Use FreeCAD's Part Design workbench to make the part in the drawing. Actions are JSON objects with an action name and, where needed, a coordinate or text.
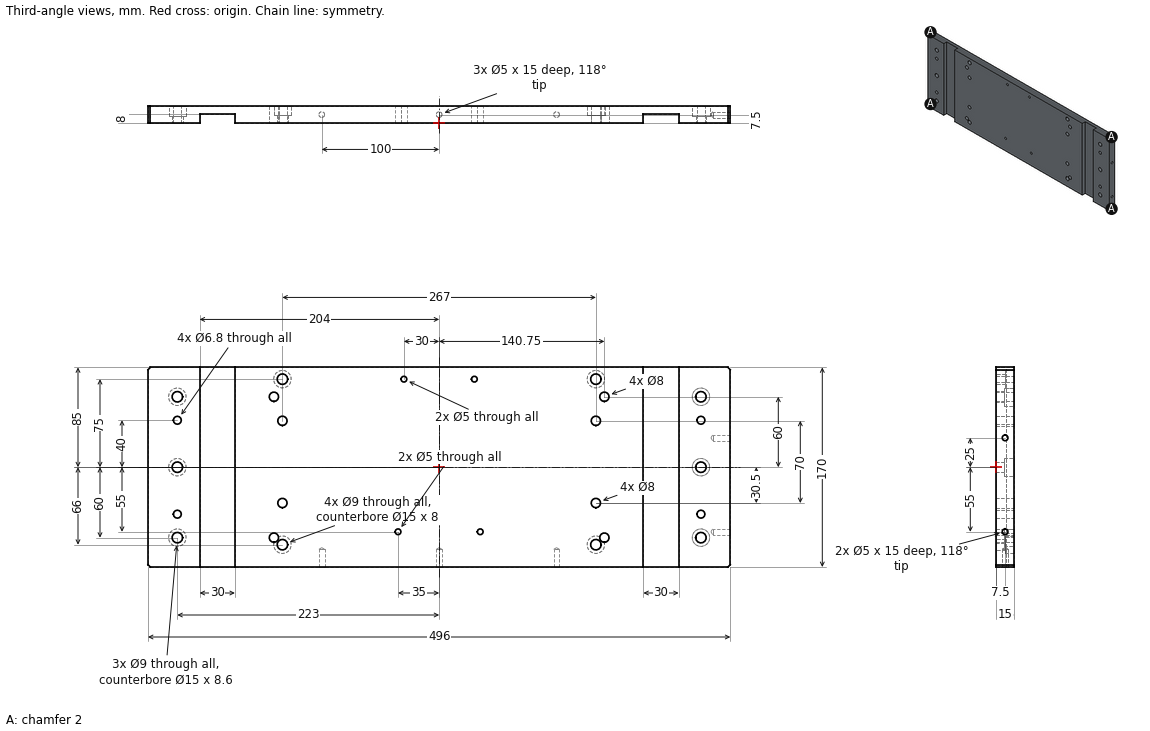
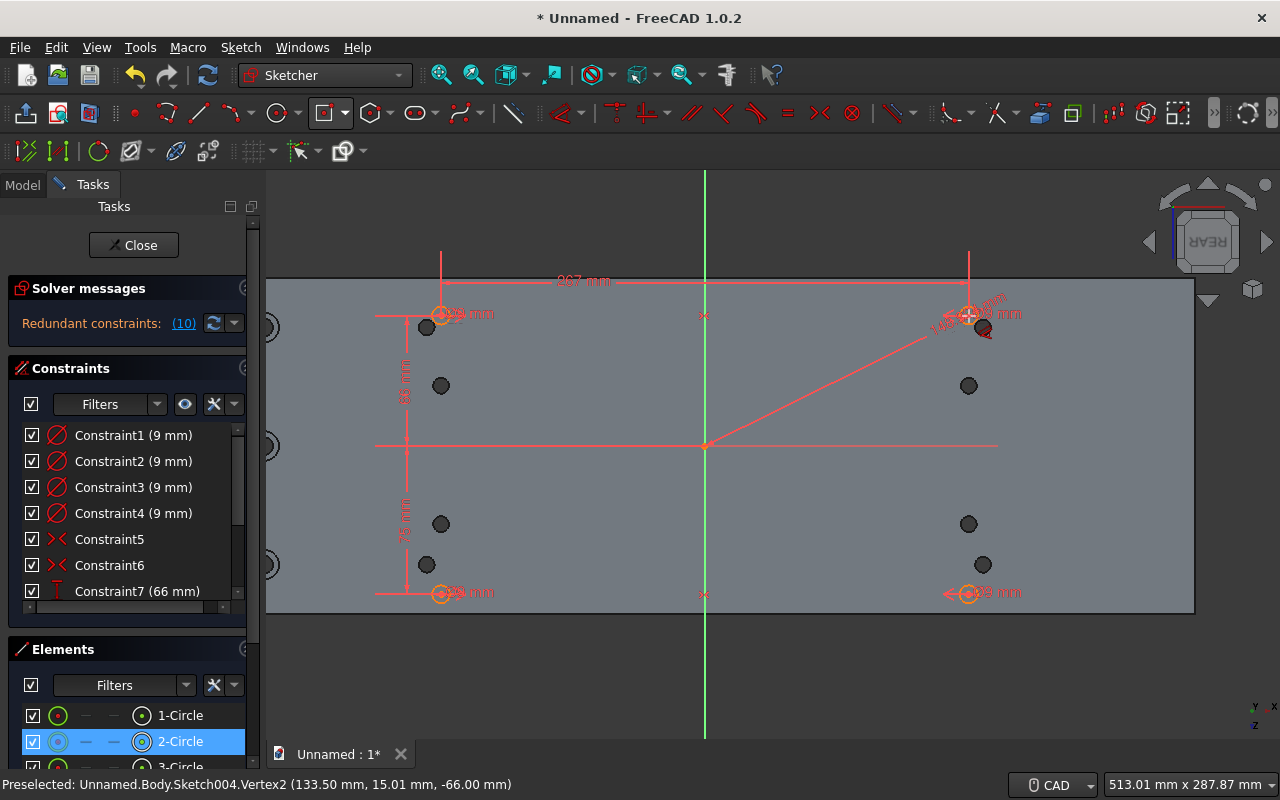
{"action": "left_click", "coordinate": [441, 594]}
{"action": "left_click", "coordinate": [584, 628]}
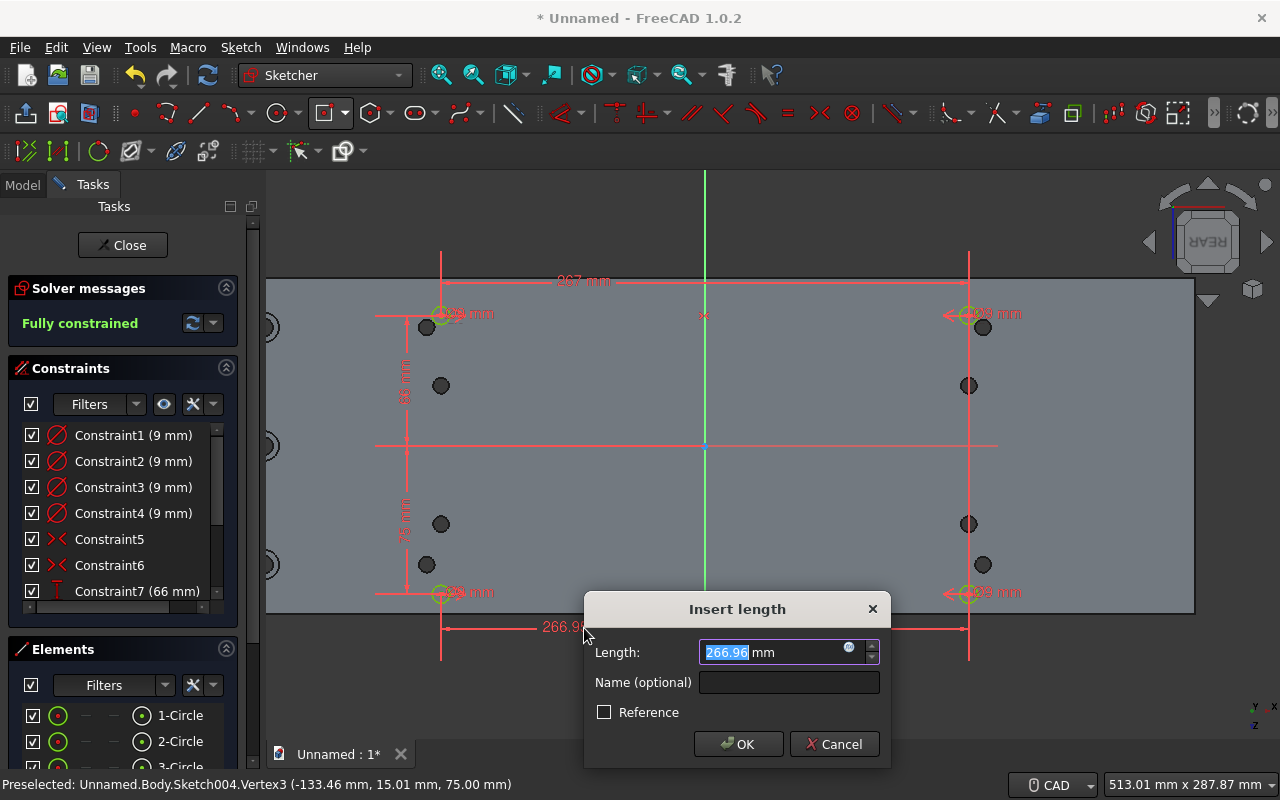
{"action": "type", "text": "267"}
{"action": "key", "text": "Return"}
{"action": "key", "text": "Escape"}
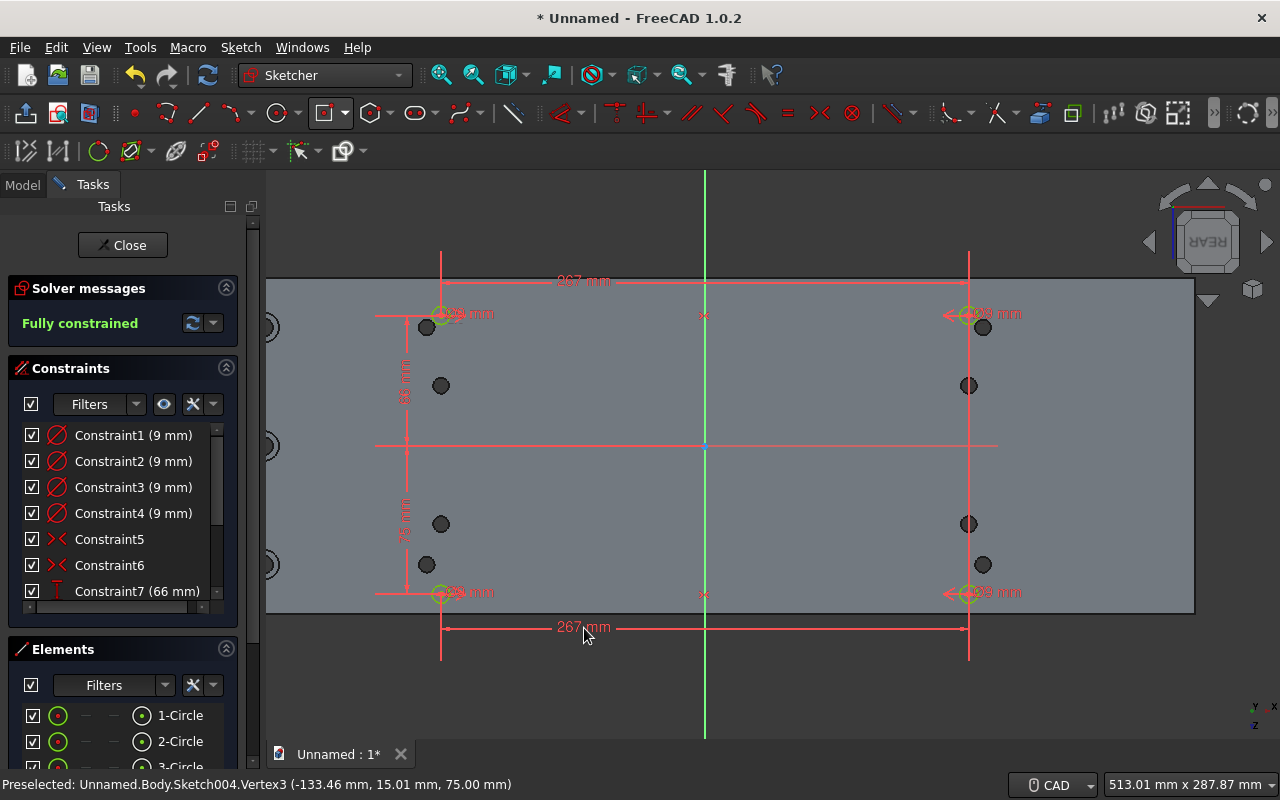
{"action": "left_click", "coordinate": [123, 245]}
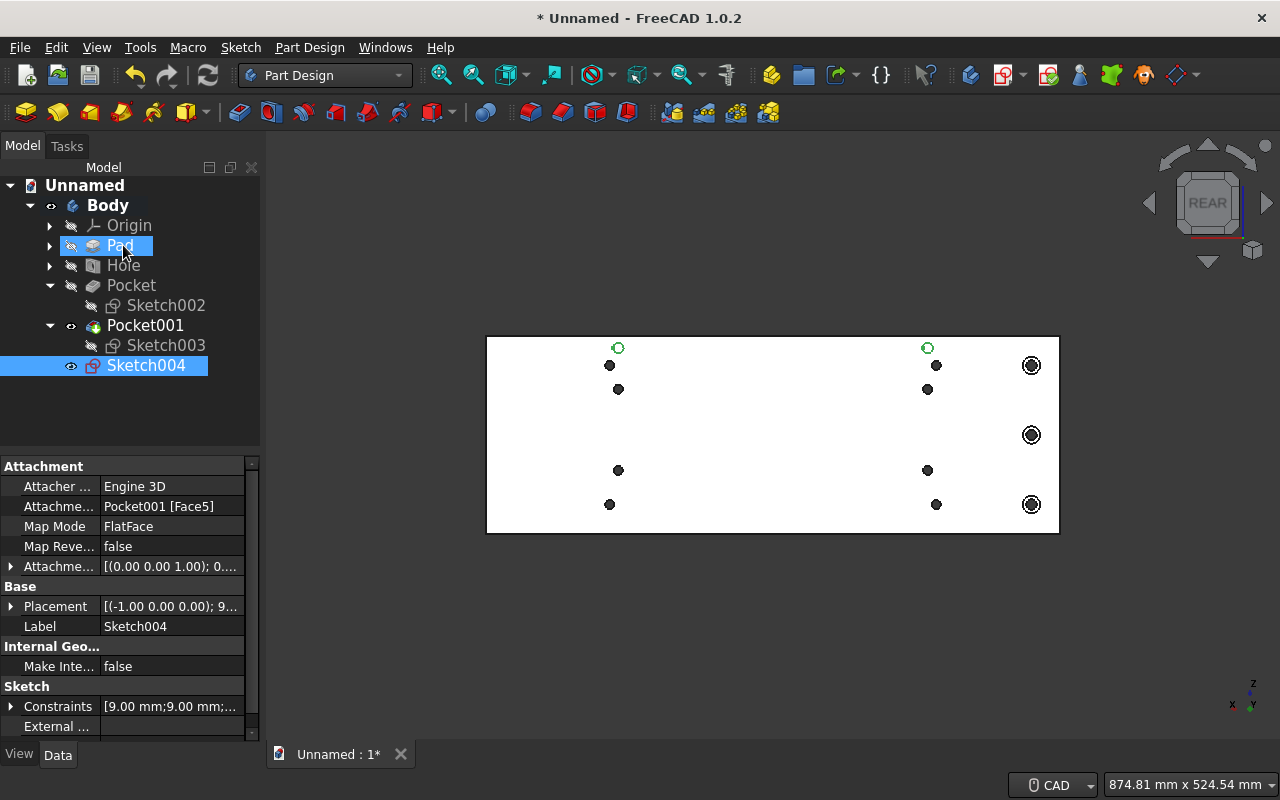
{"action": "left_click", "coordinate": [272, 112]}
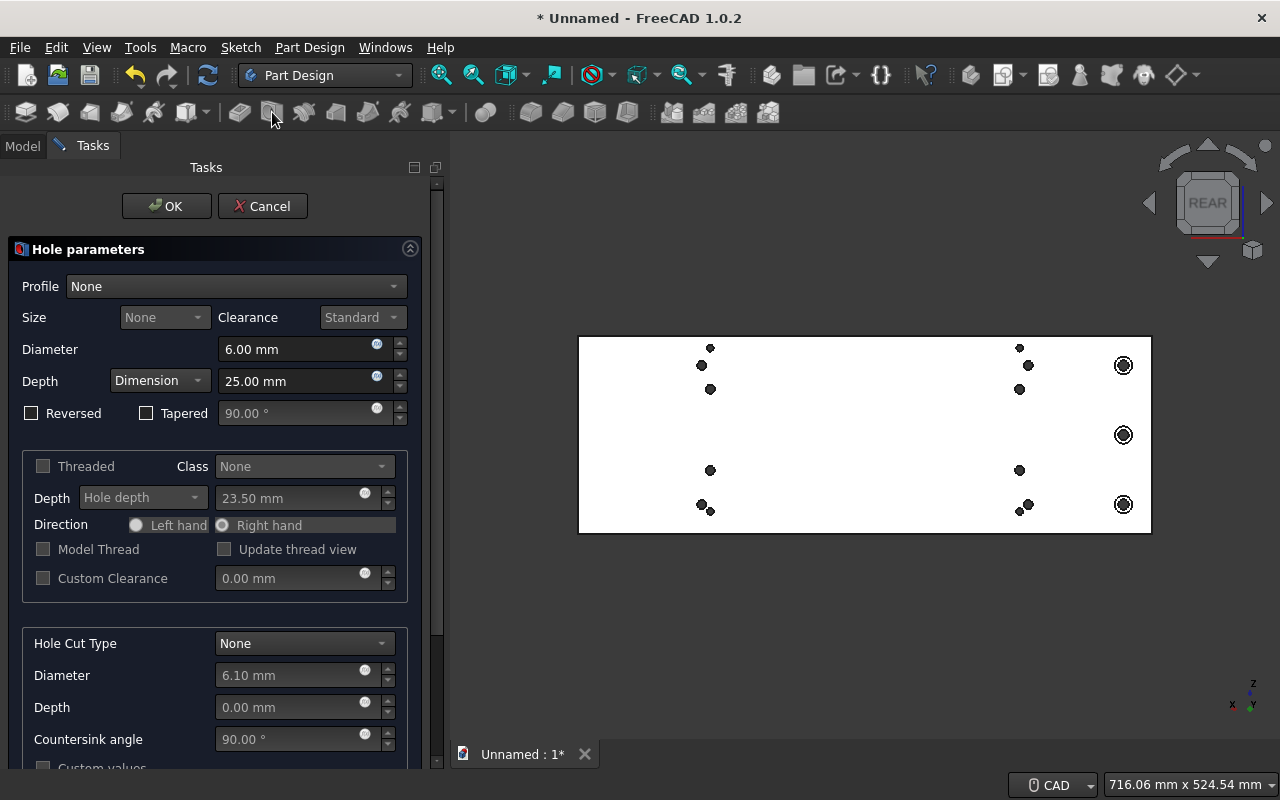
{"action": "triple_click", "coordinate": [305, 349]}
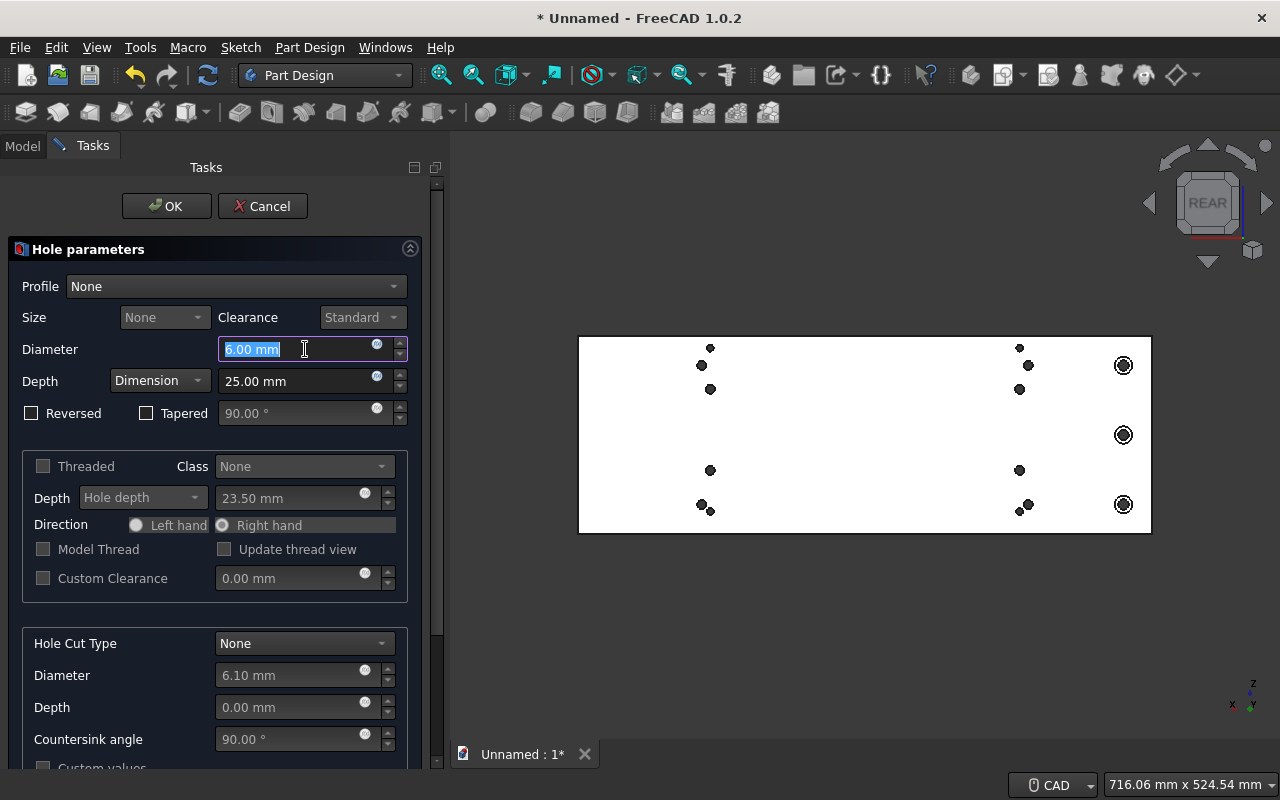
{"action": "type", "text": "9"}
{"action": "key", "text": "Tab"}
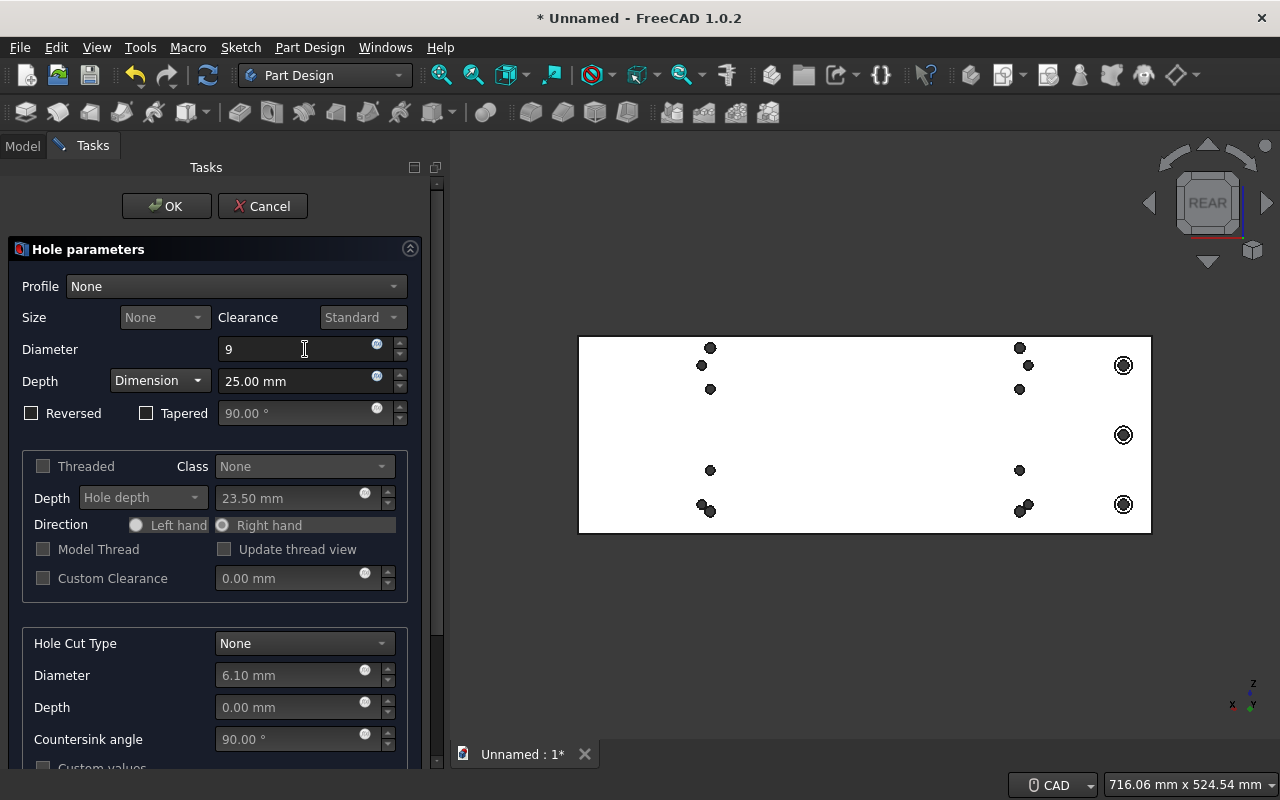
{"action": "left_click", "coordinate": [161, 380]}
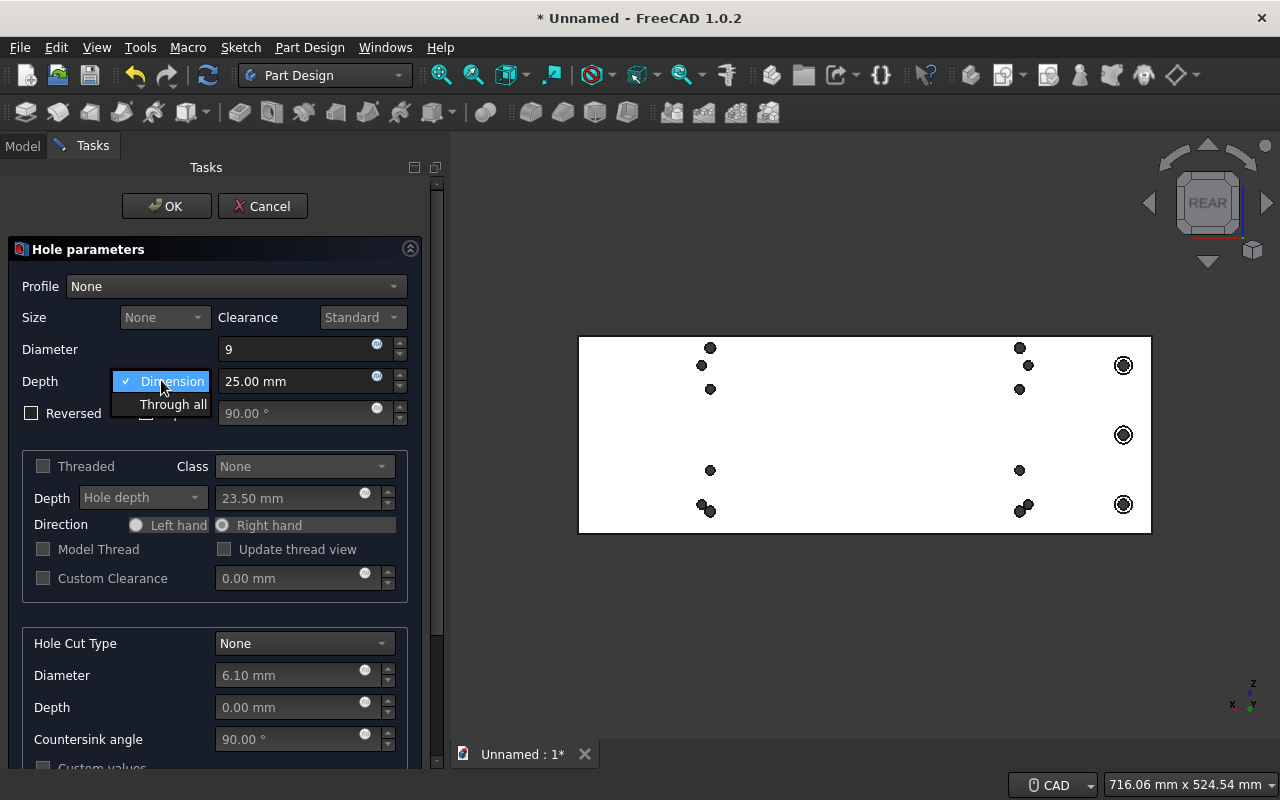
{"action": "left_click", "coordinate": [160, 404]}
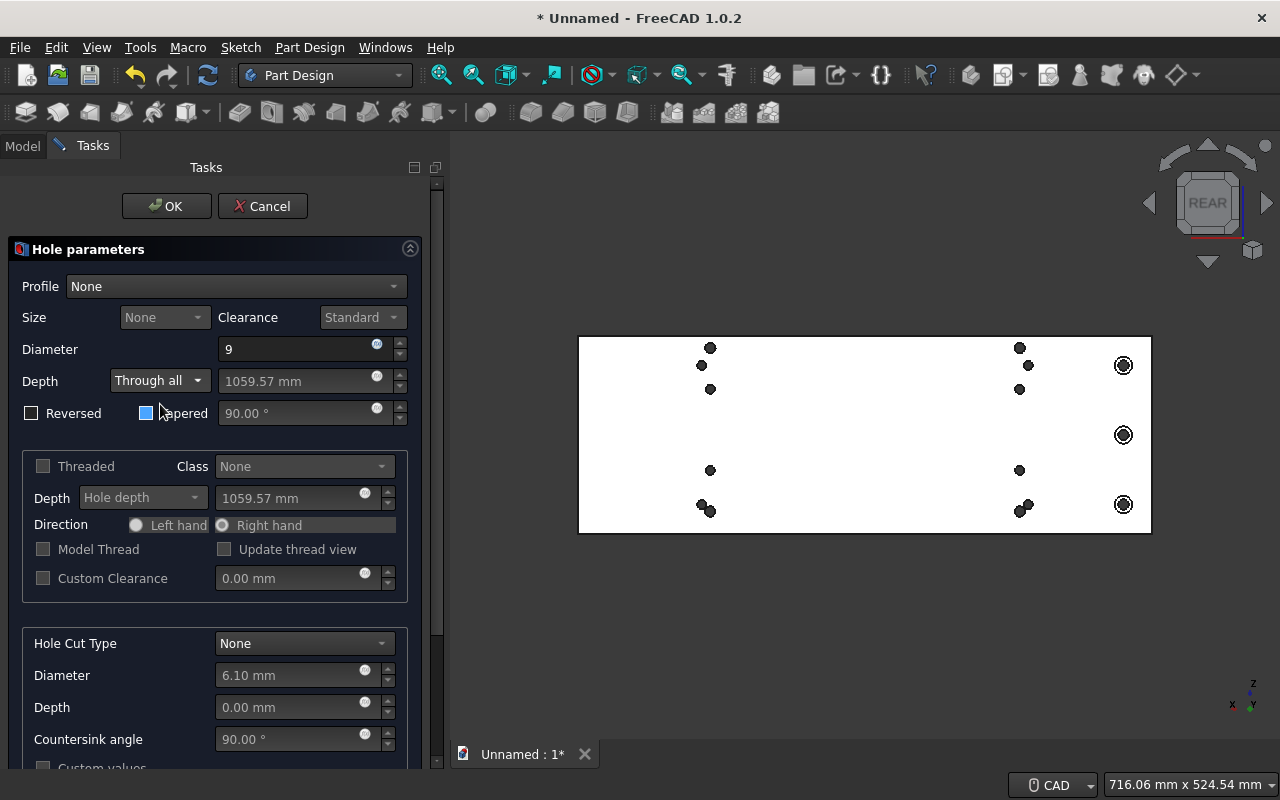
{"action": "left_click", "coordinate": [306, 644]}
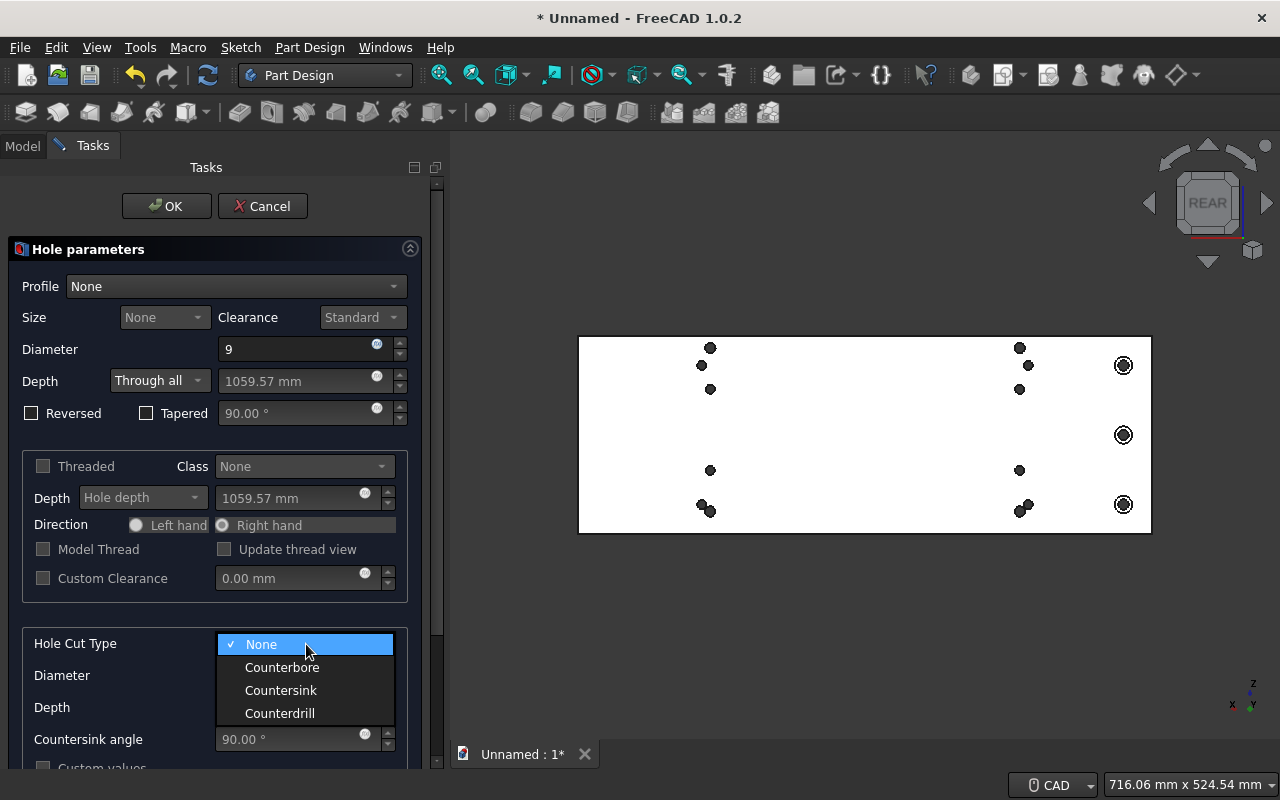
{"action": "left_click", "coordinate": [304, 668]}